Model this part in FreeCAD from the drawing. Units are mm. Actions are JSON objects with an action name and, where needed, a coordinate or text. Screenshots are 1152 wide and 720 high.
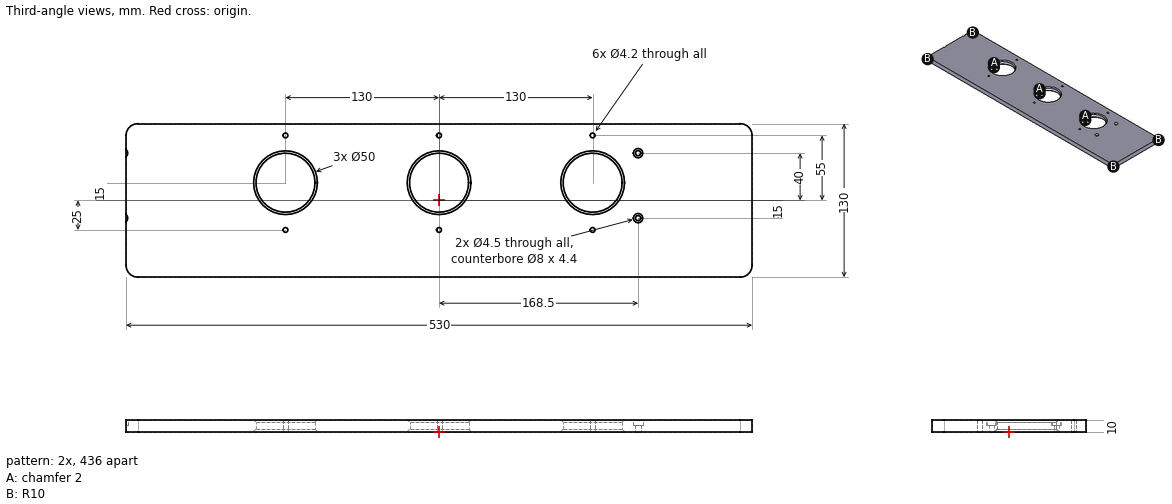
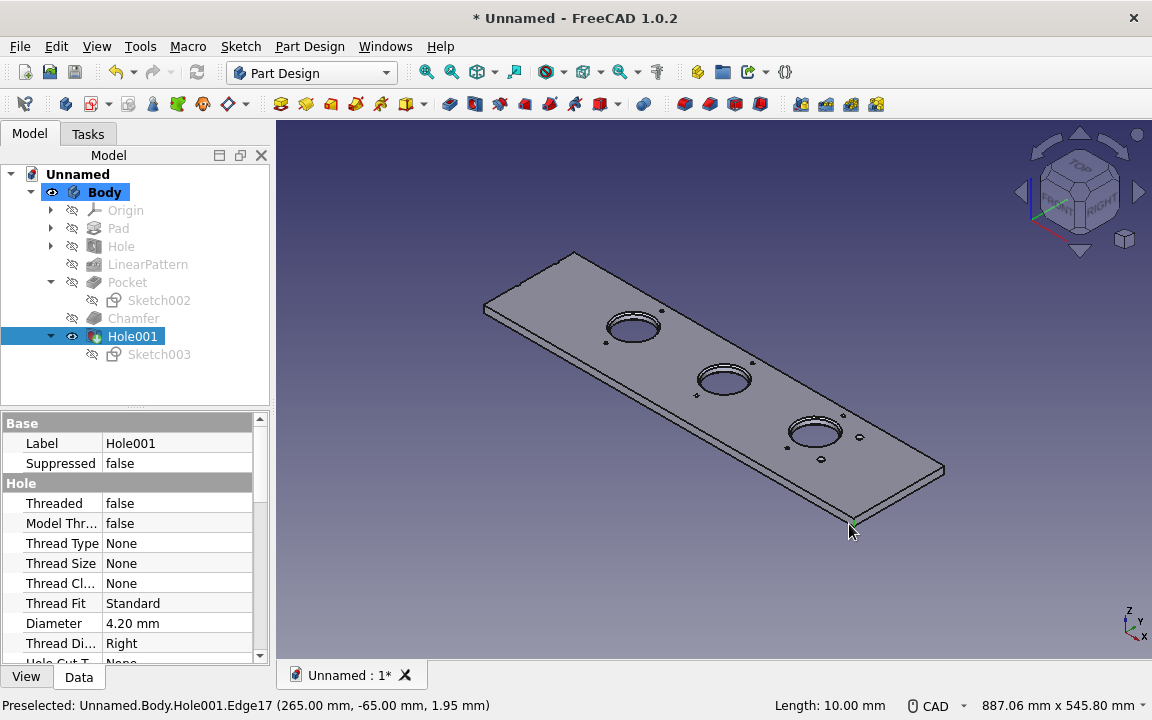
{"action": "scroll", "coordinate": [484, 308], "scroll_direction": "up", "scroll_amount": 7}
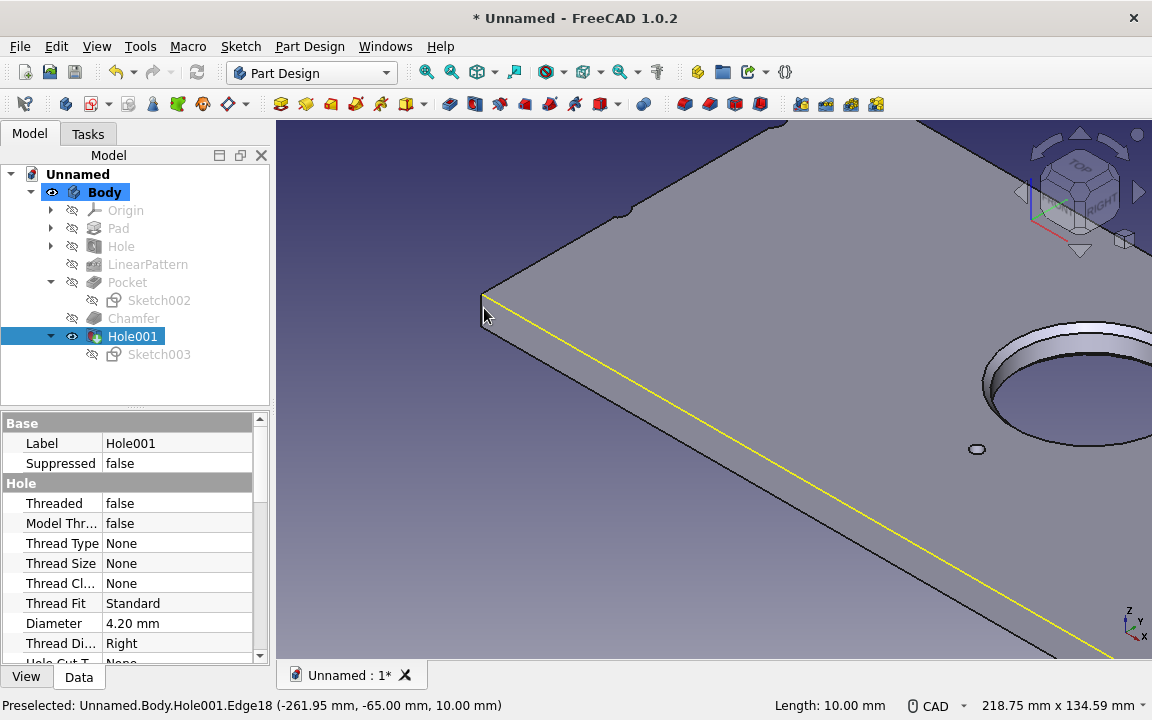
{"action": "left_click", "coordinate": [427, 72]}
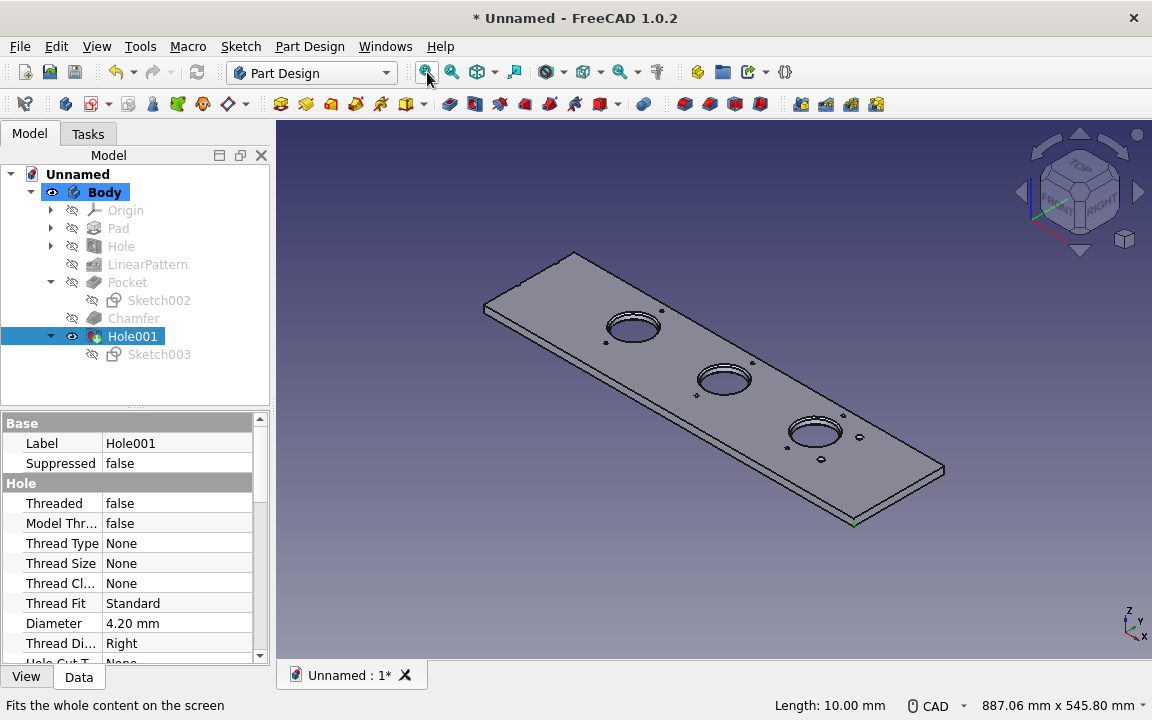
{"action": "key", "text": "2"}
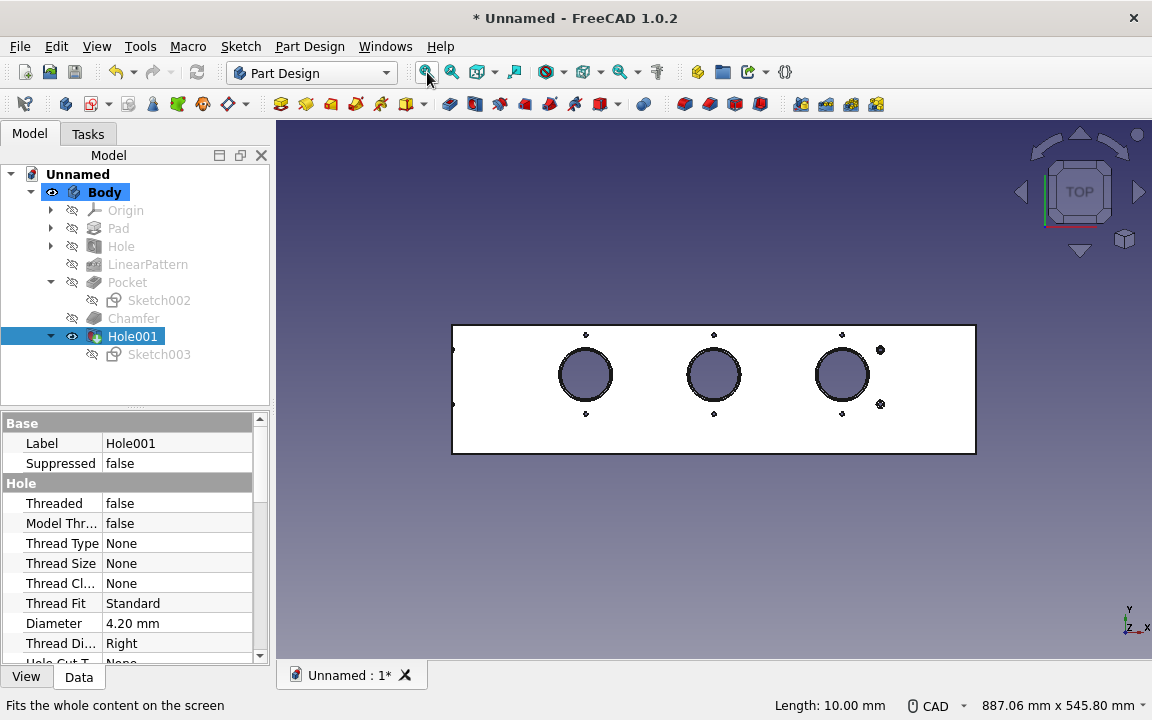
{"action": "scroll", "coordinate": [452, 453], "scroll_direction": "up", "scroll_amount": 7}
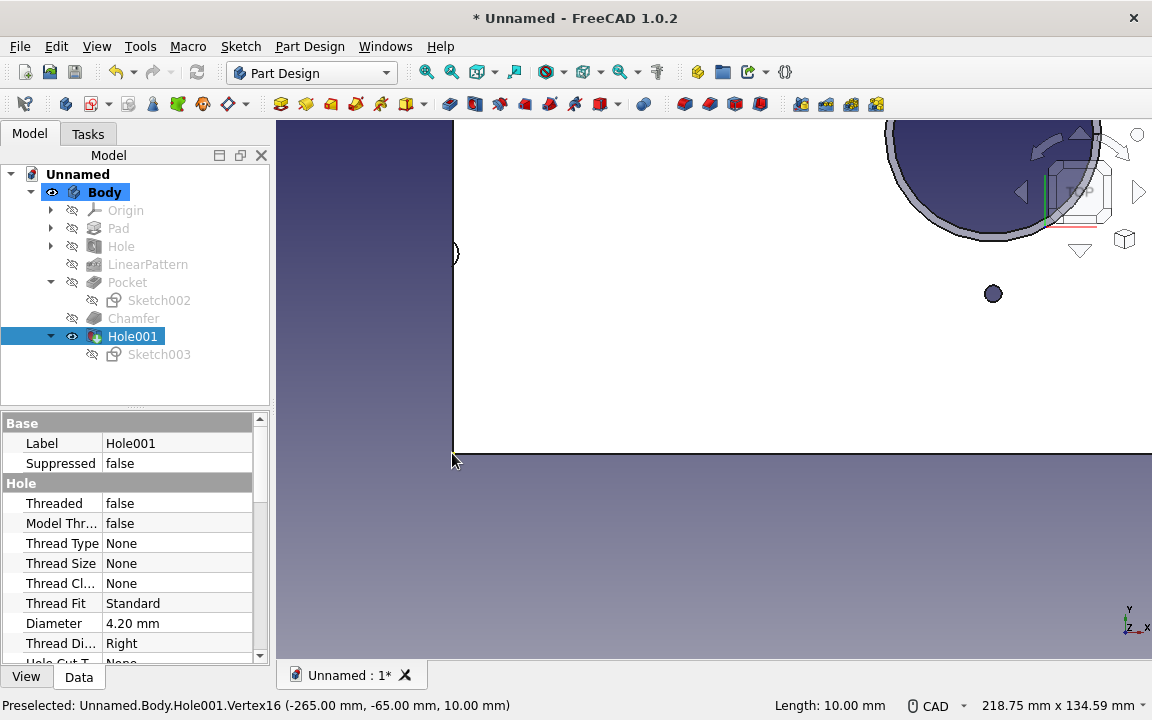
{"action": "left_click", "coordinate": [427, 72]}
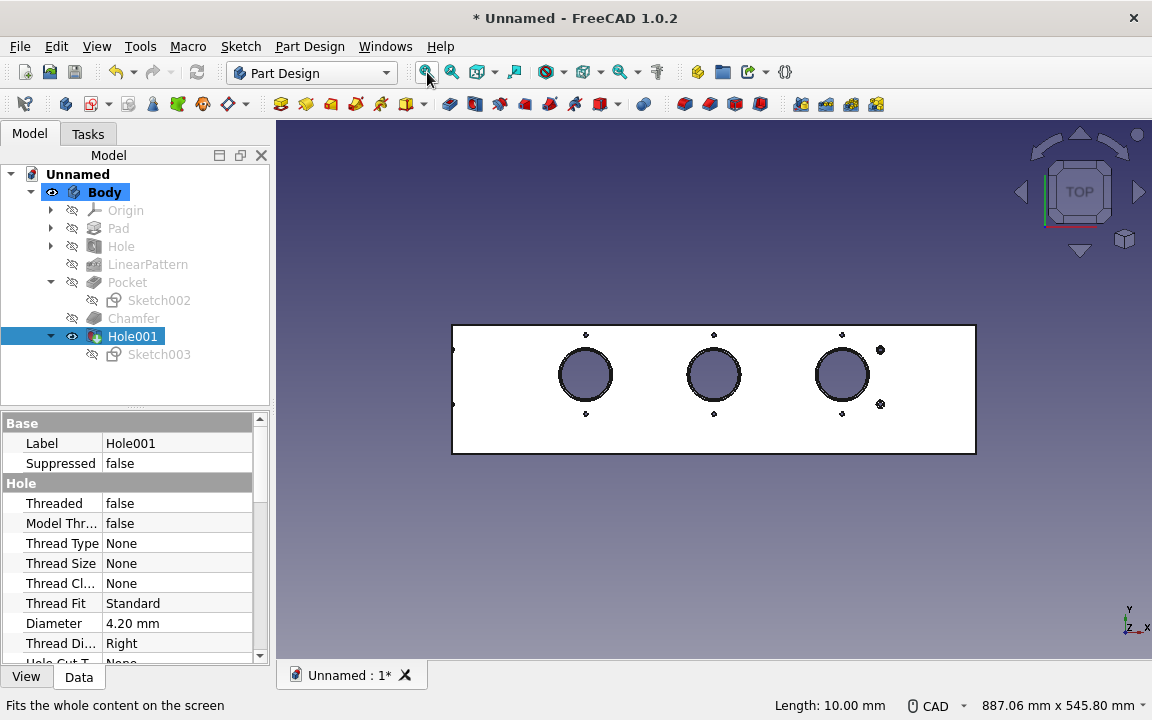
{"action": "key", "text": "0"}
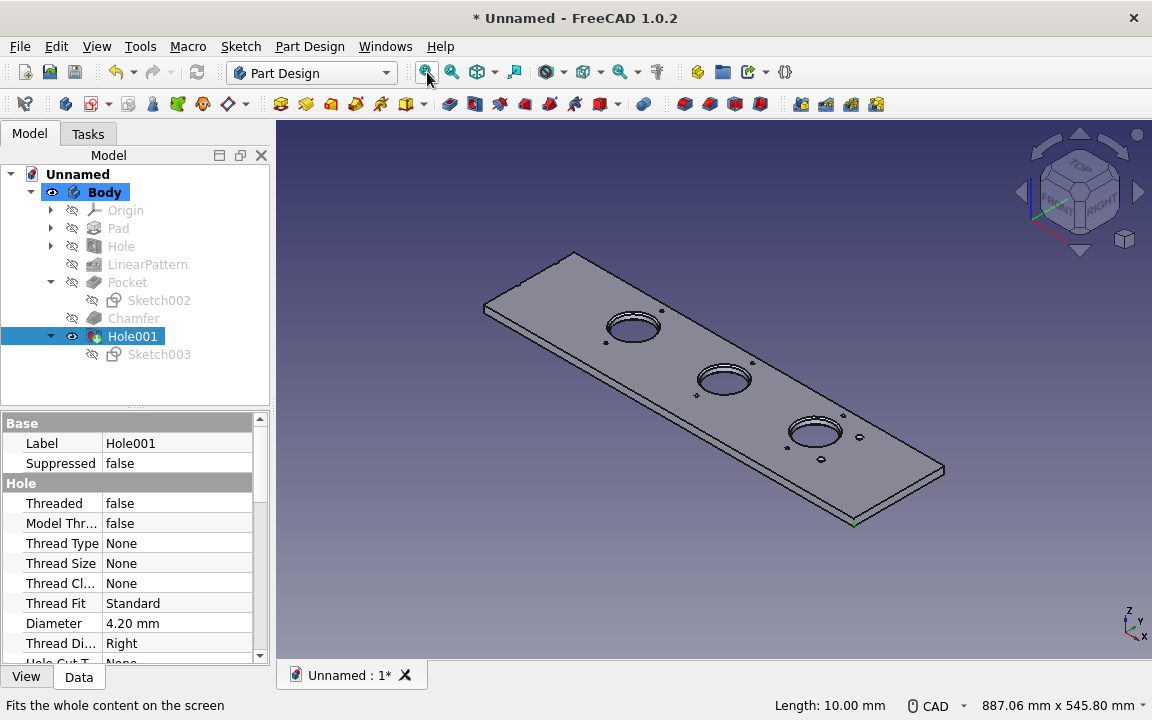
{"action": "scroll", "coordinate": [484, 308], "scroll_direction": "up", "scroll_amount": 7}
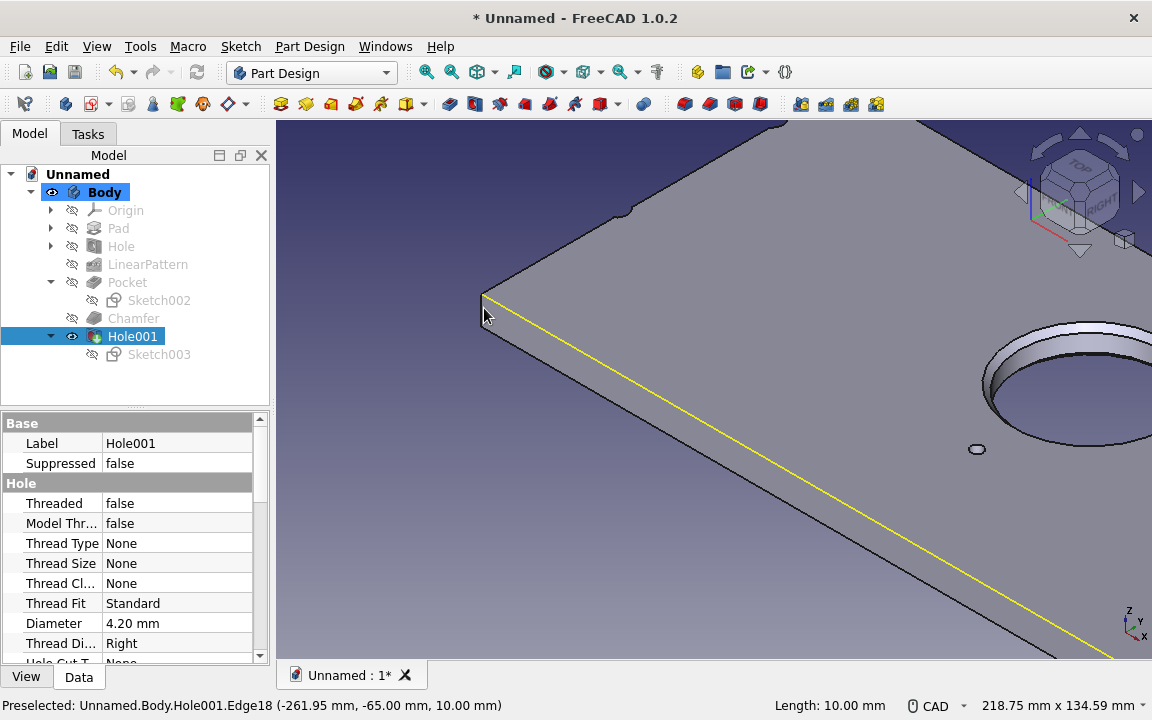
{"action": "left_click", "coordinate": [427, 72]}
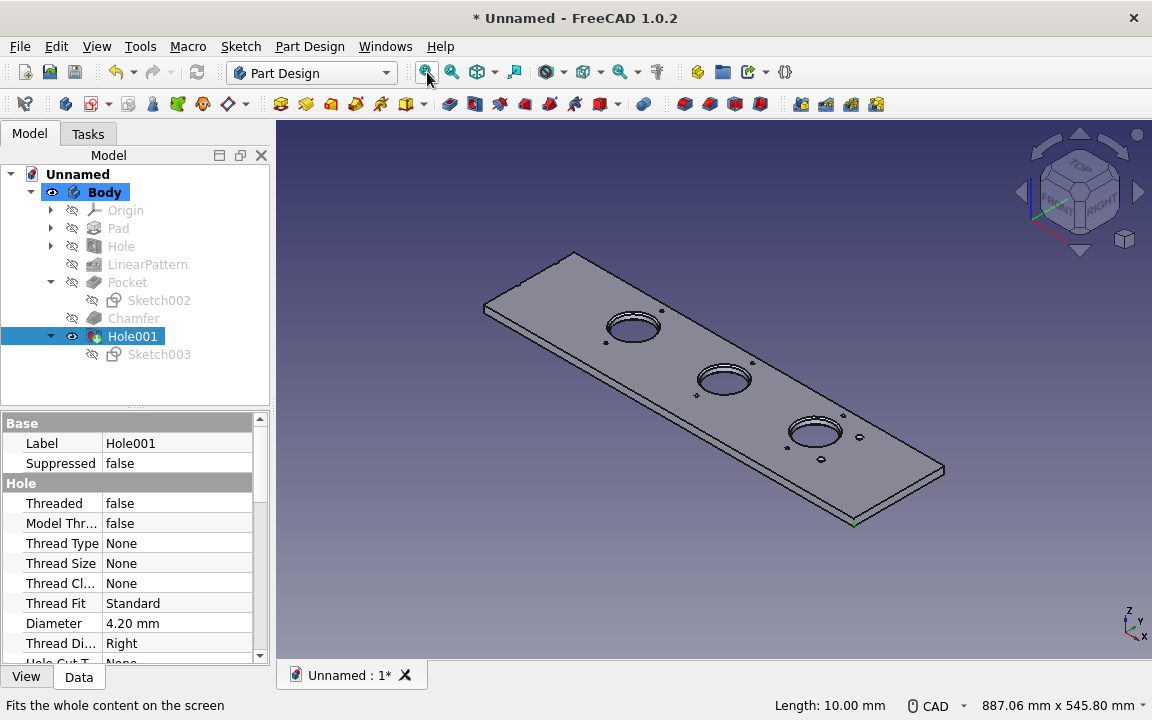
{"action": "key", "text": "1"}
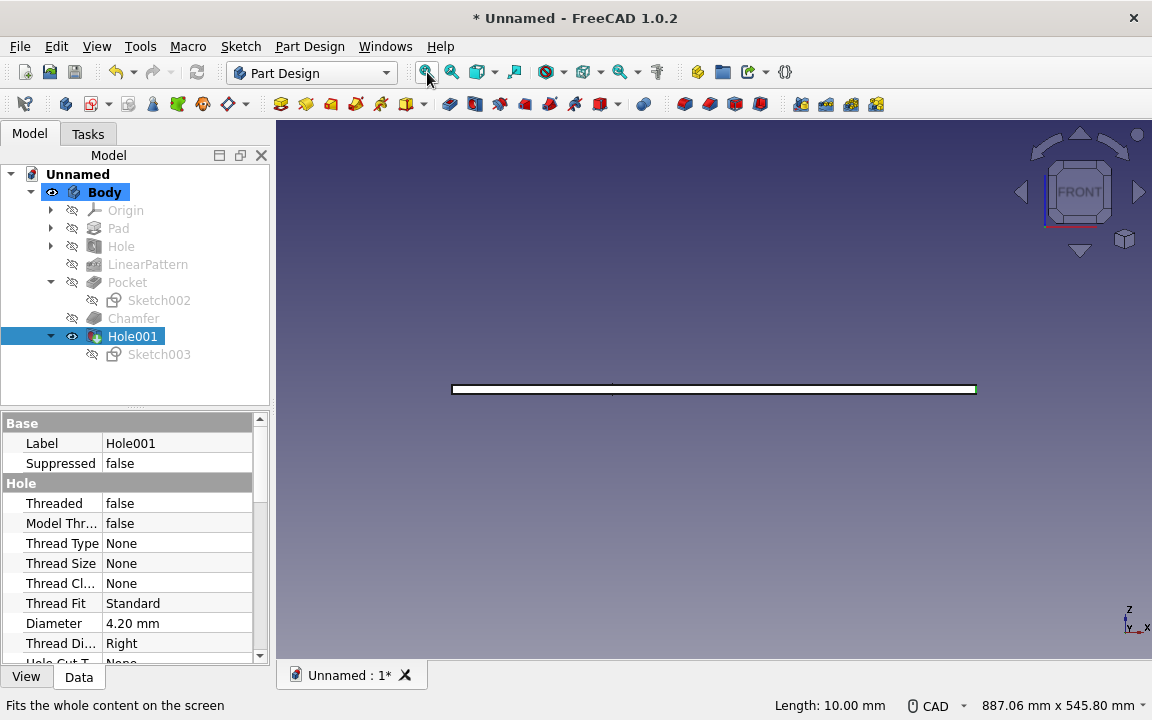
{"action": "scroll", "coordinate": [452, 388], "scroll_direction": "up", "scroll_amount": 7}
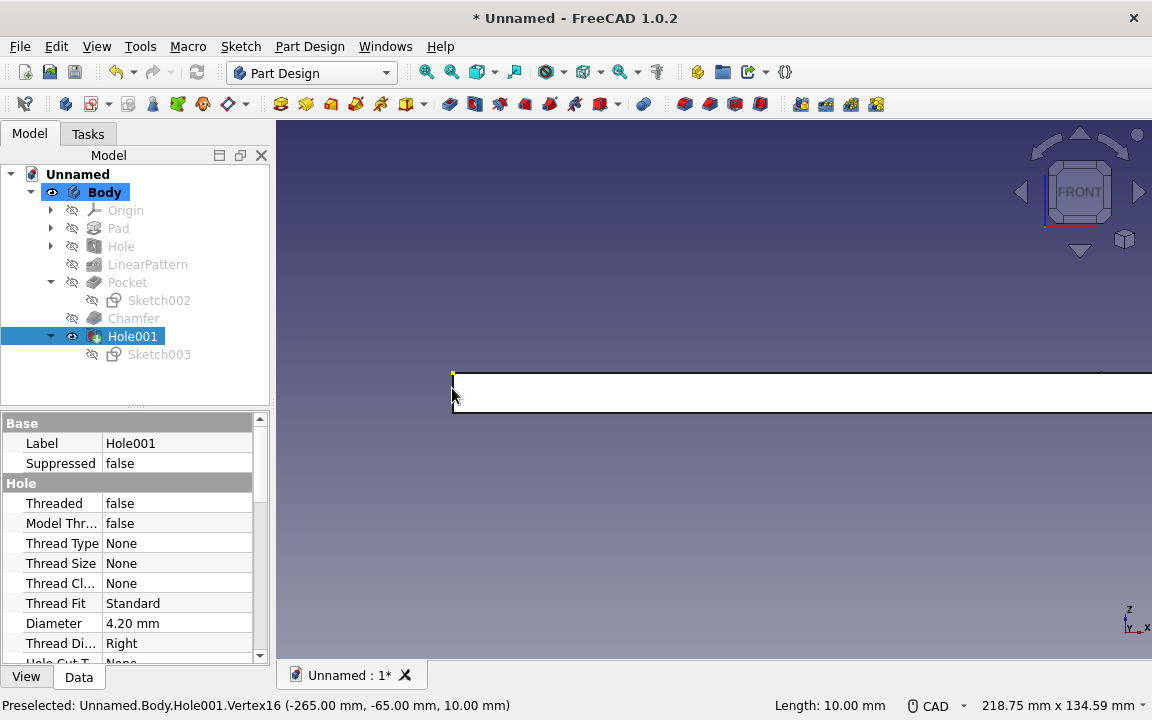
{"action": "left_click", "coordinate": [453, 392], "text": "ctrl"}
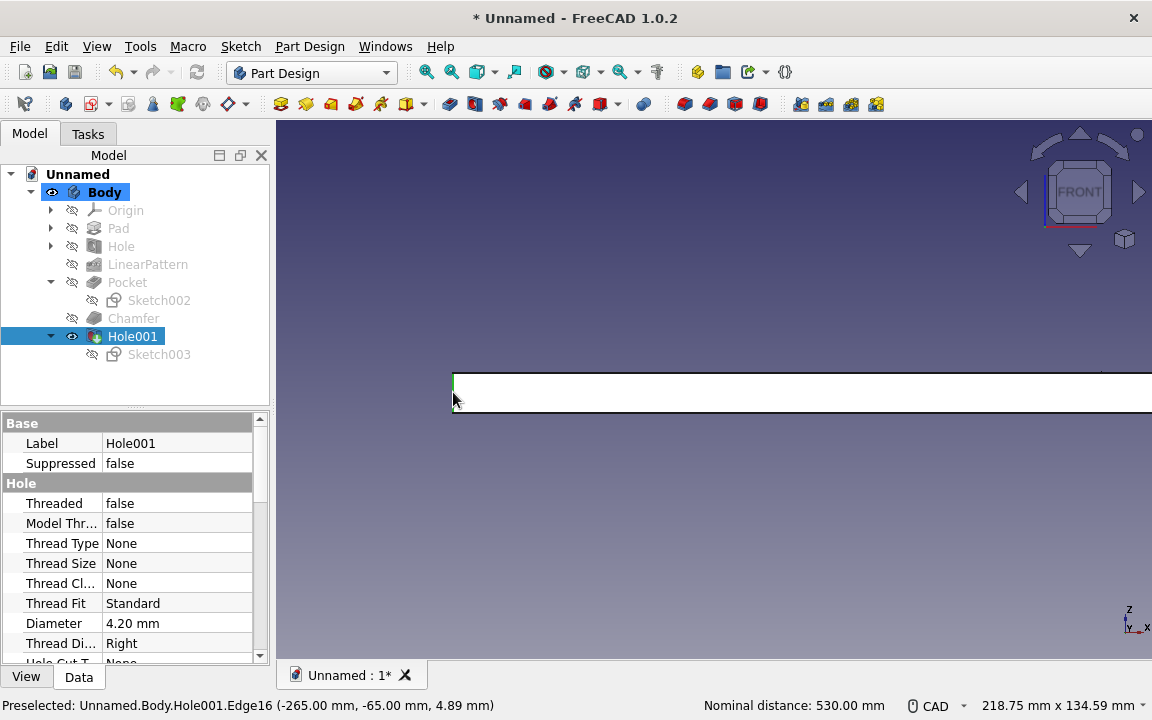
{"action": "key", "text": "v f"}